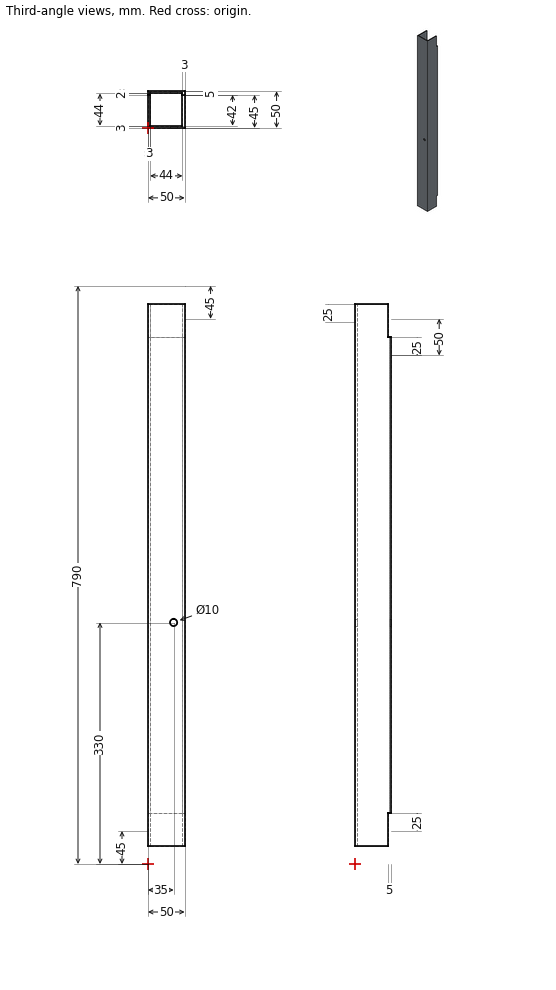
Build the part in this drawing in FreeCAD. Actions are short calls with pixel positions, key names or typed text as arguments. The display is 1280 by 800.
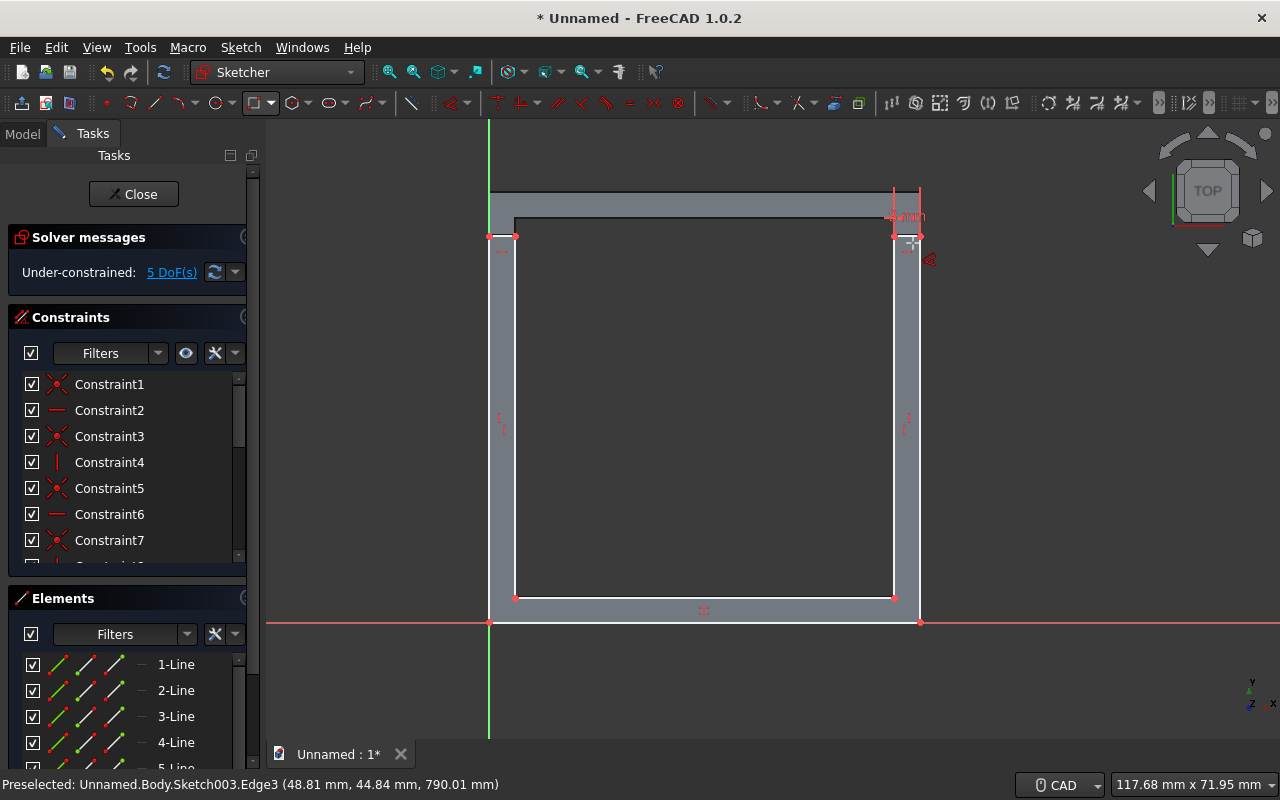
scroll(508, 236, up, 3)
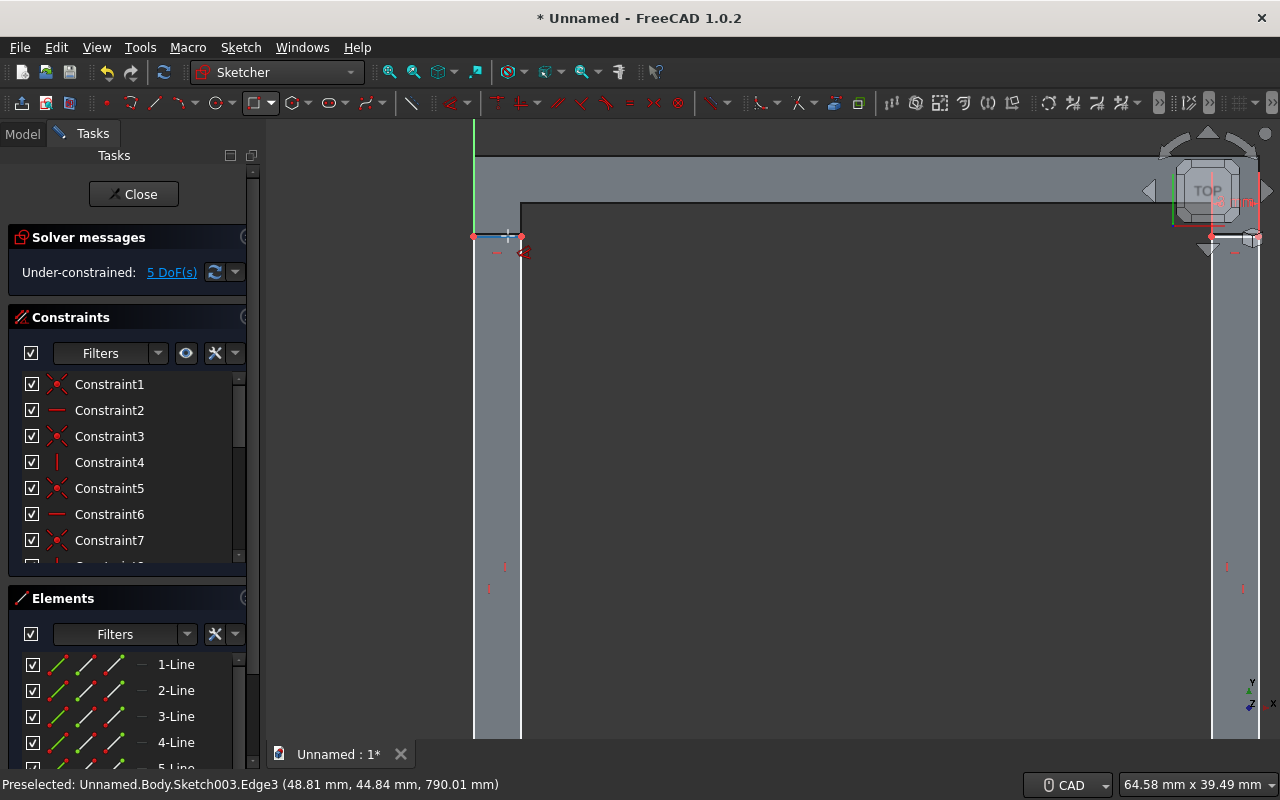
click(507, 237)
click(497, 203)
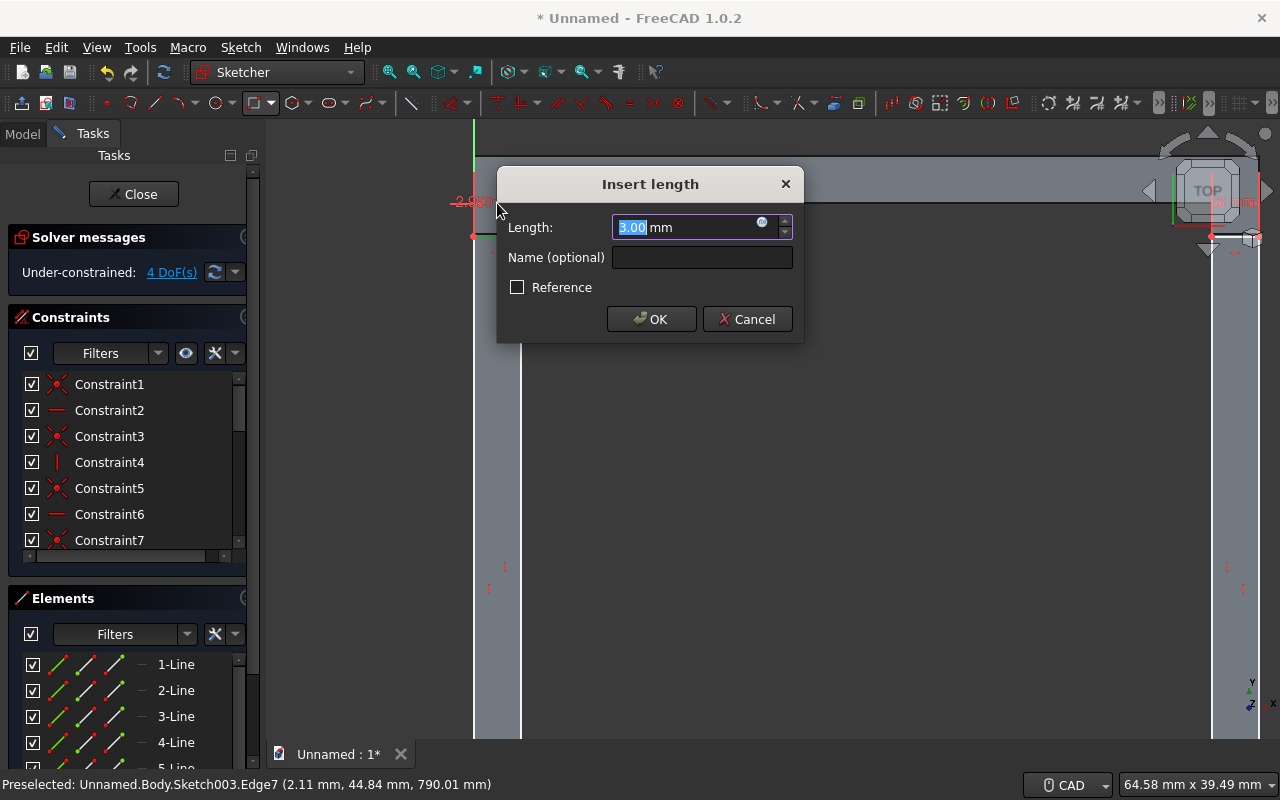
text(3)
key(Return)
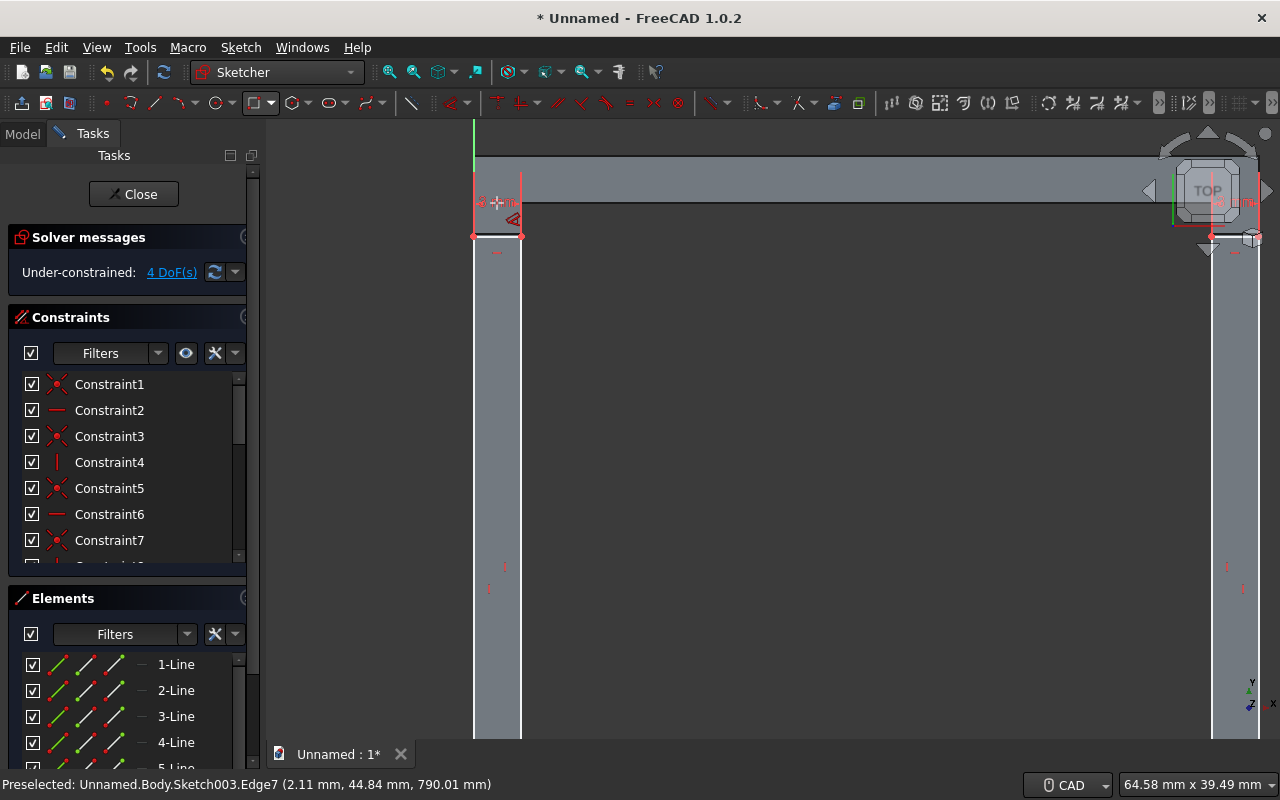
scroll(508, 236, down, 3)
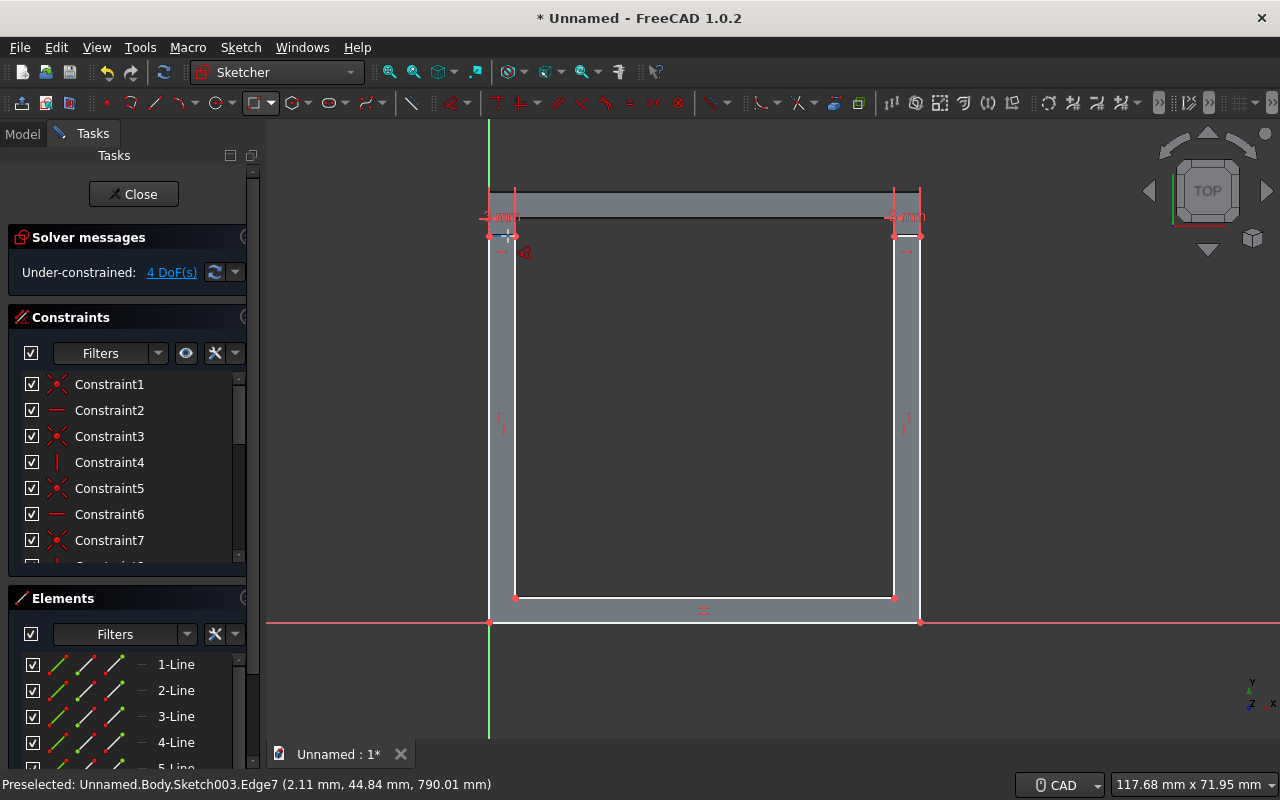
click(619, 623)
click(705, 657)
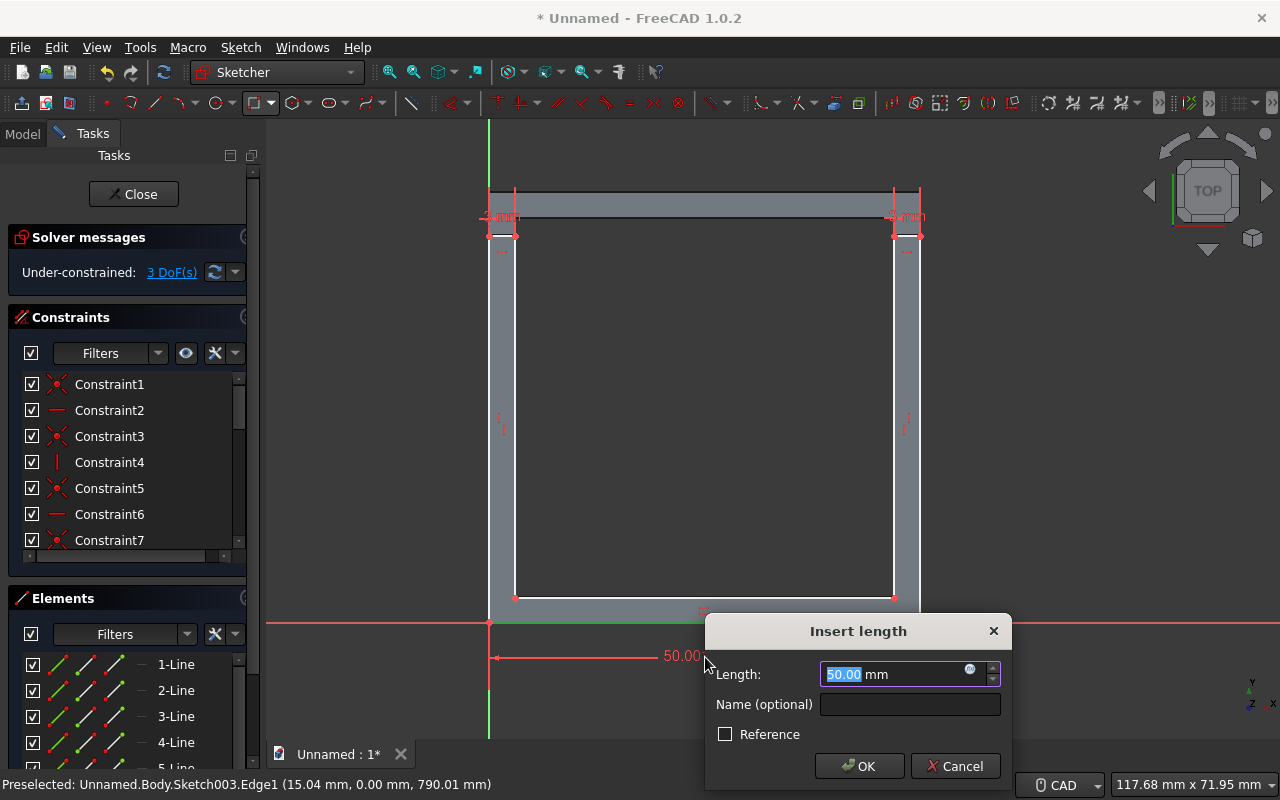
text(50)
key(Return)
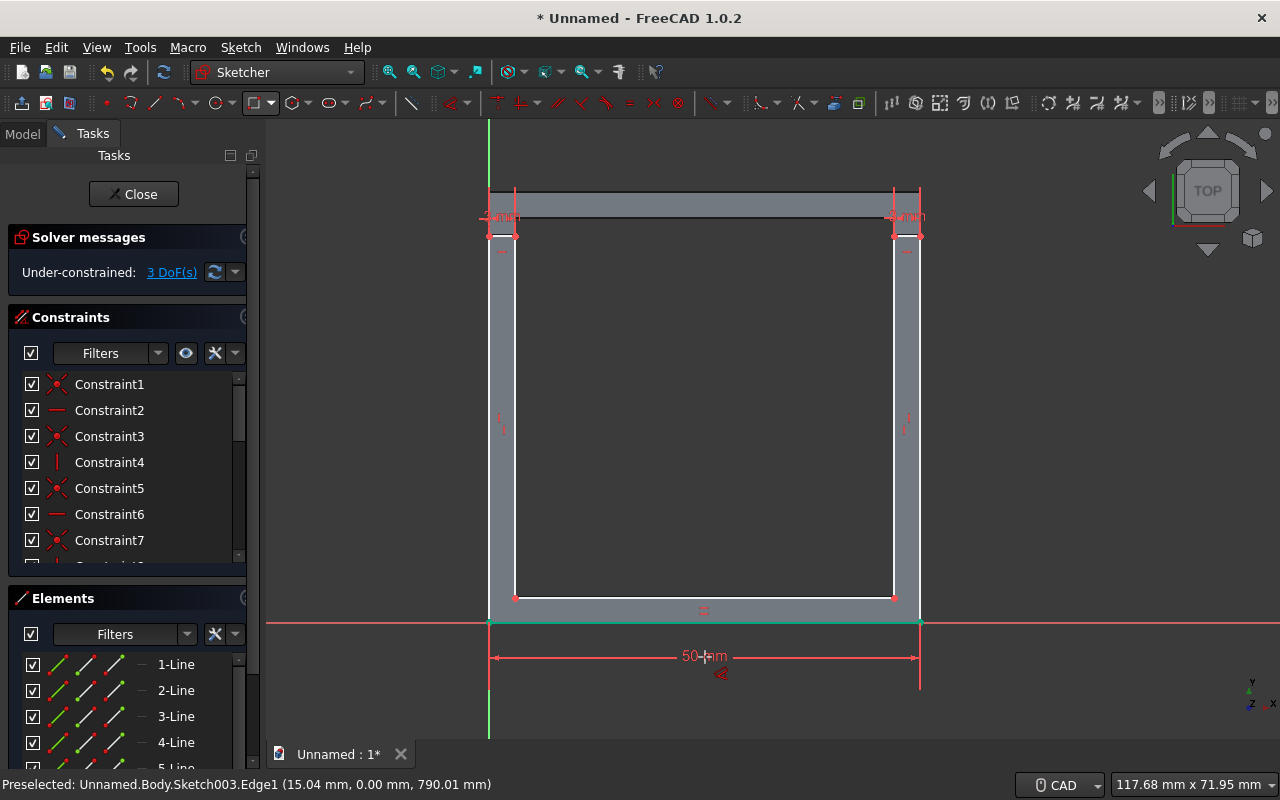
click(920, 507)
click(954, 430)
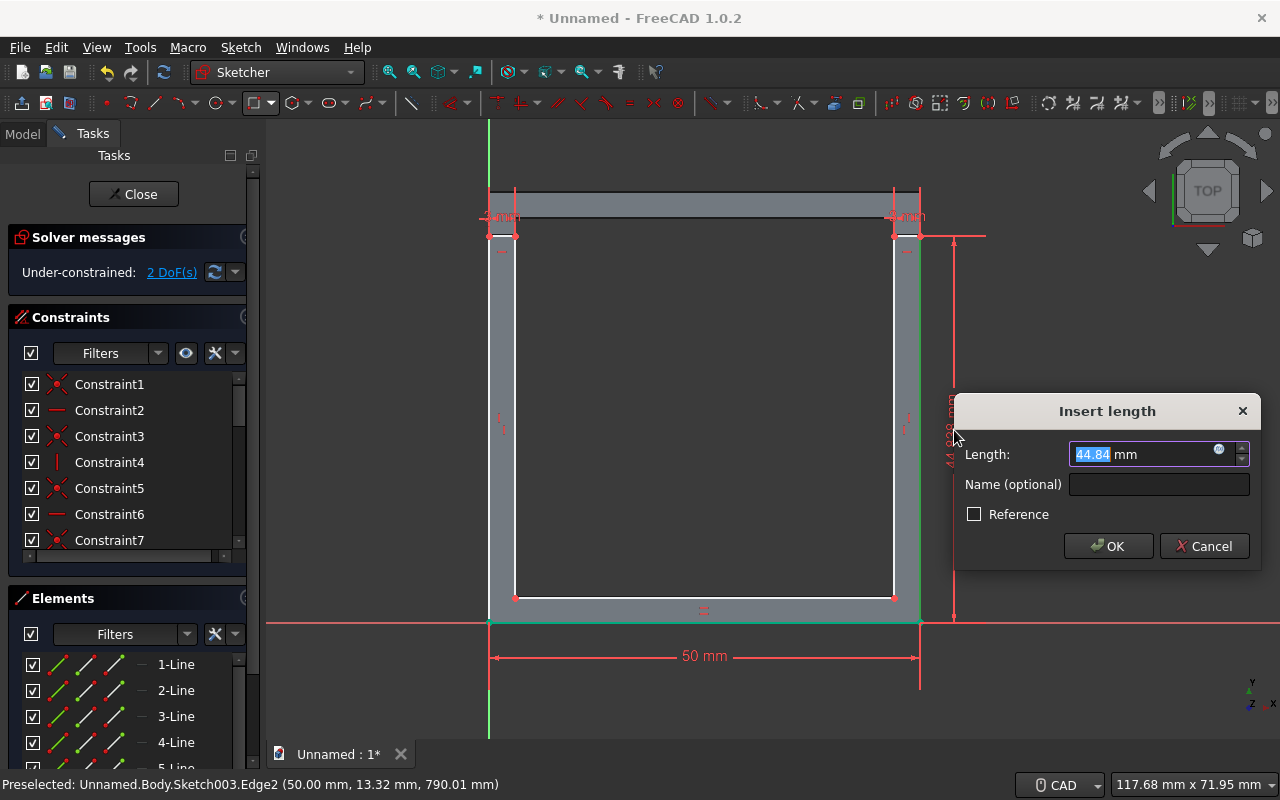
text(45)
key(Return)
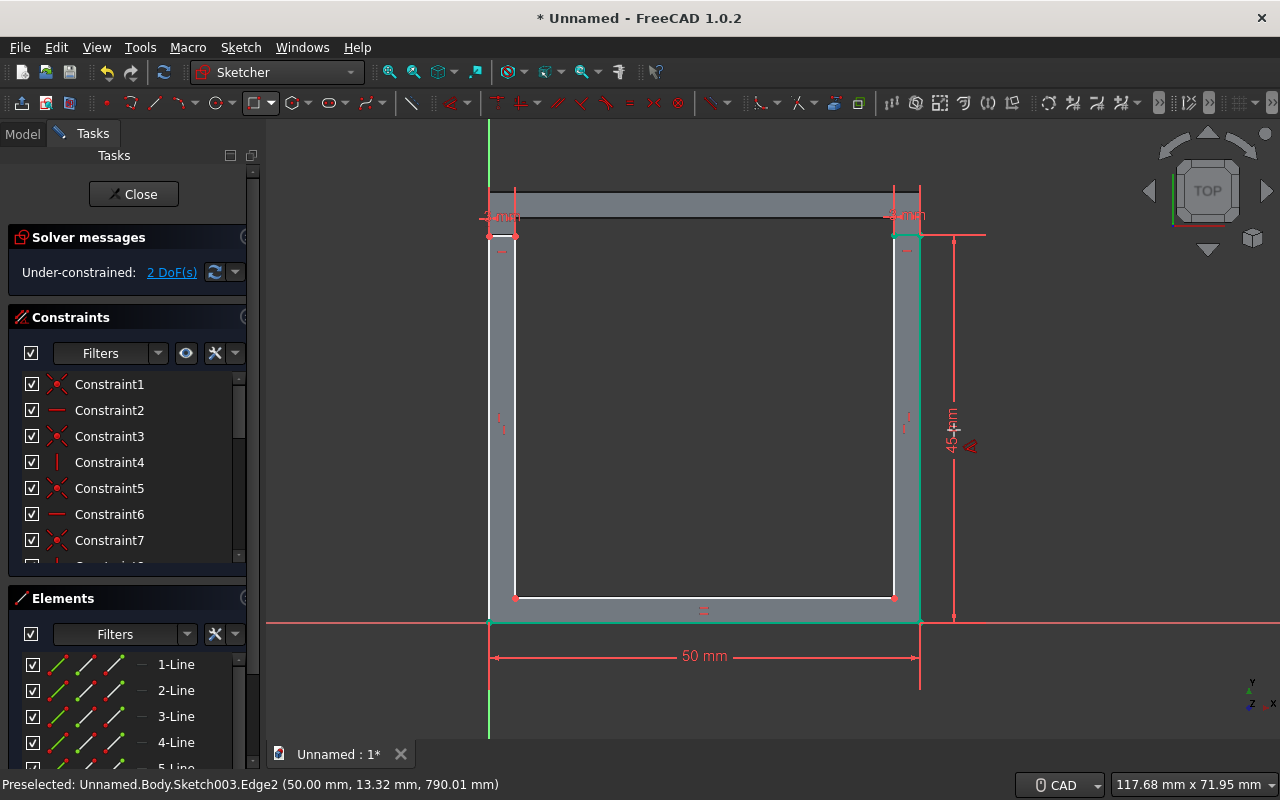
click(894, 344)
click(860, 417)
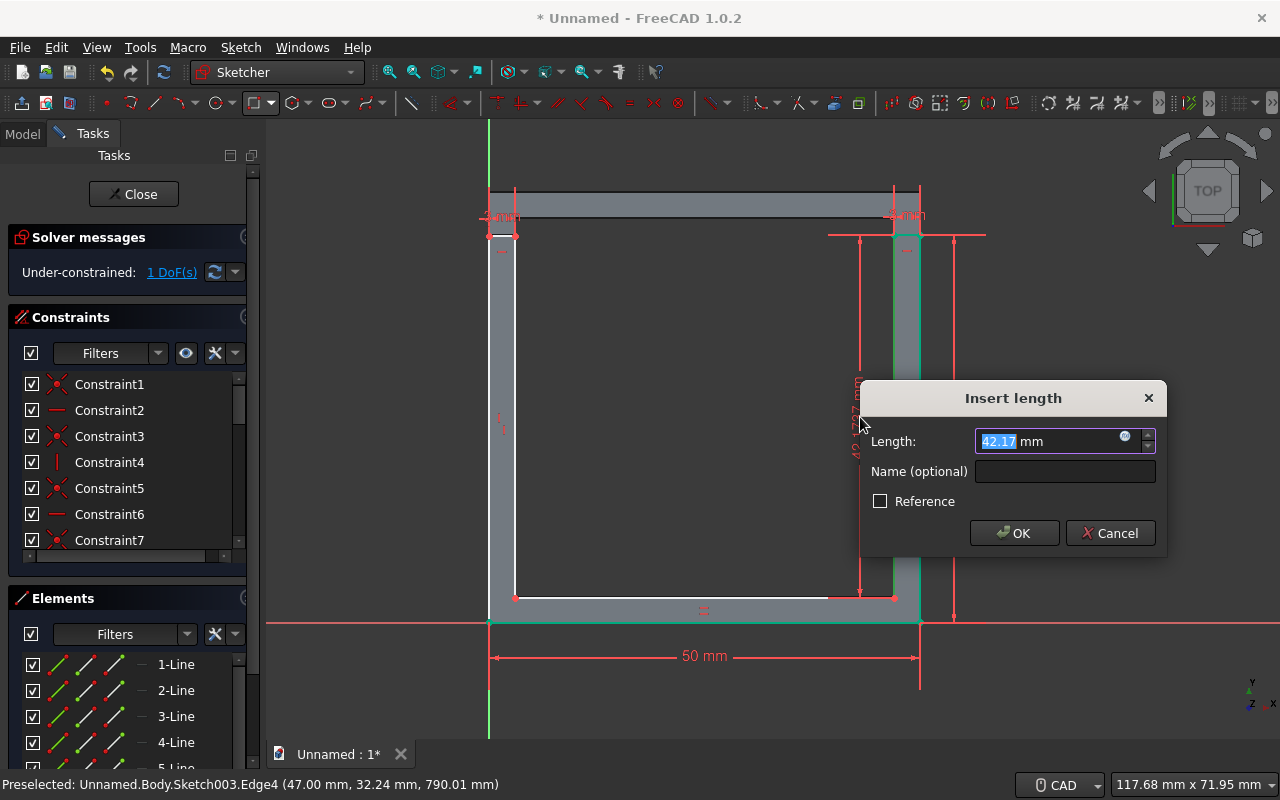
text(42)
key(Return)